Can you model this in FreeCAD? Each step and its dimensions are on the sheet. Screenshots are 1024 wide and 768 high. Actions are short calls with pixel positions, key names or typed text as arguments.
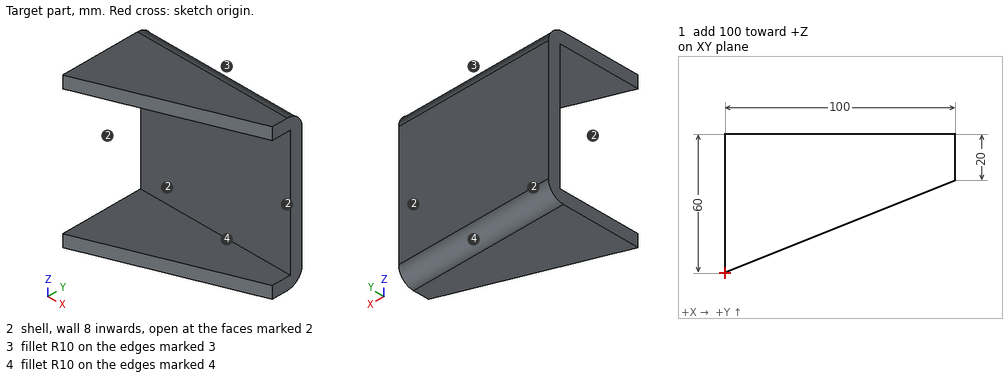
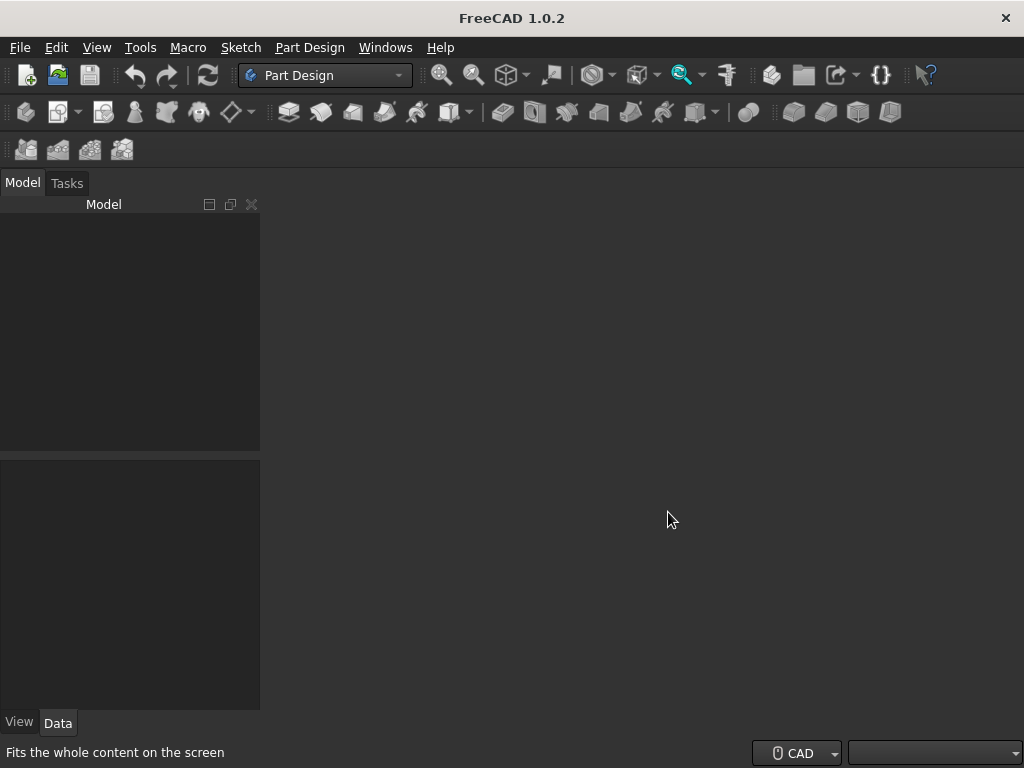
click(26, 76)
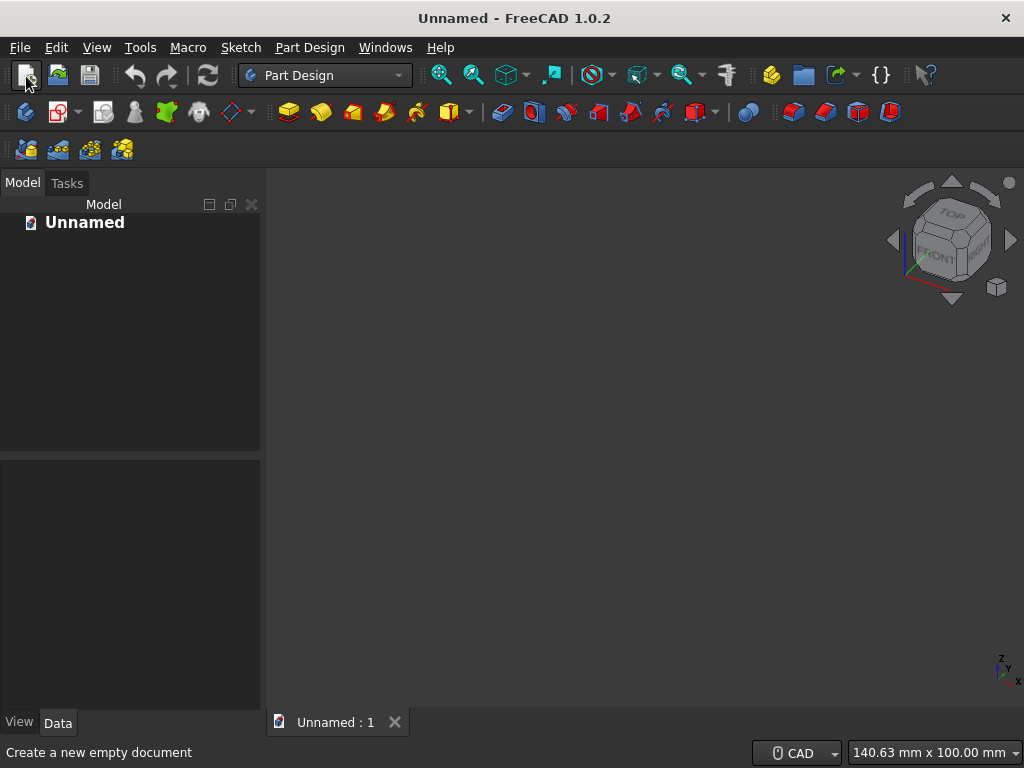
click(58, 112)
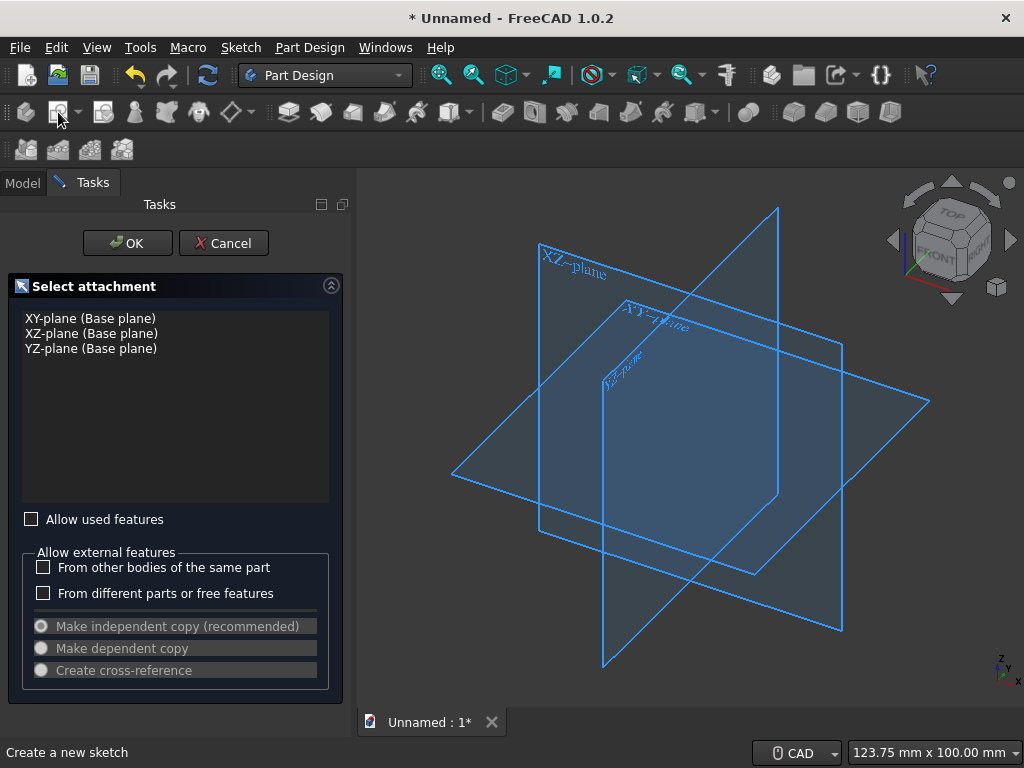
click(82, 318)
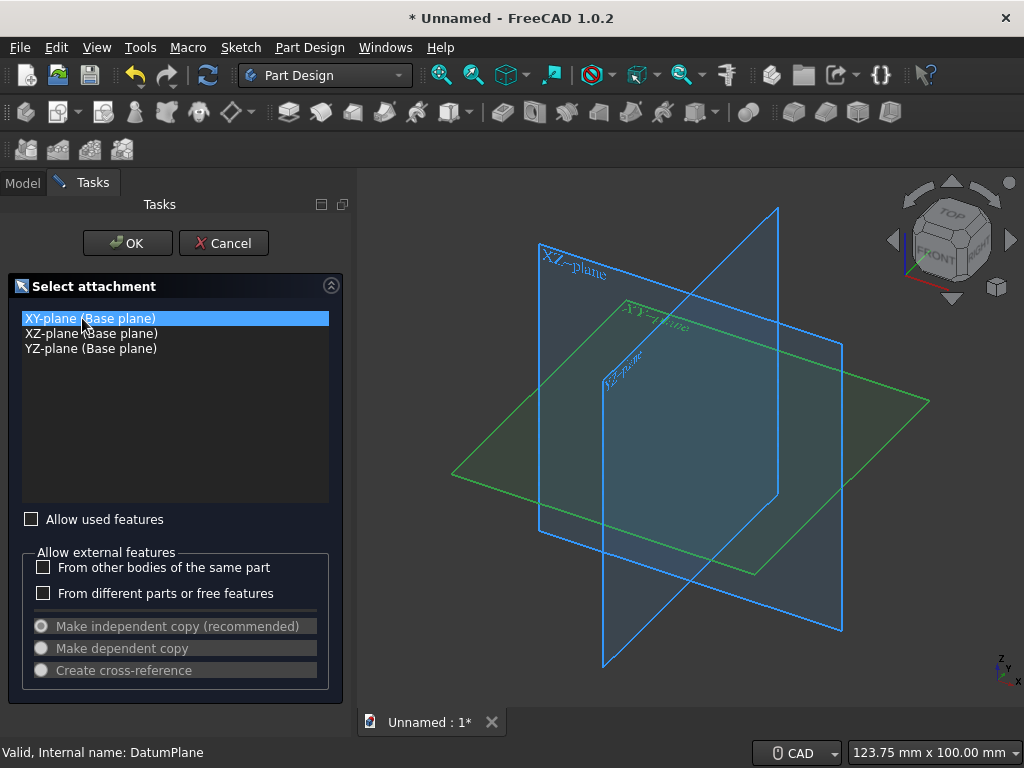
click(128, 243)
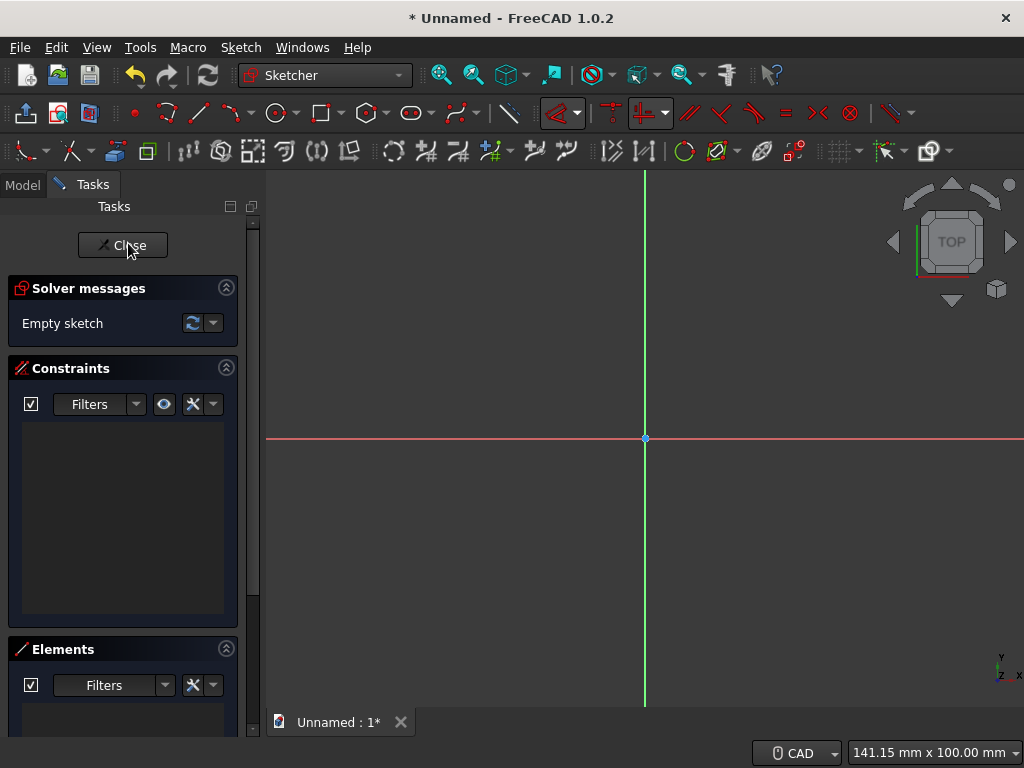
scroll(294, 634, down, 3)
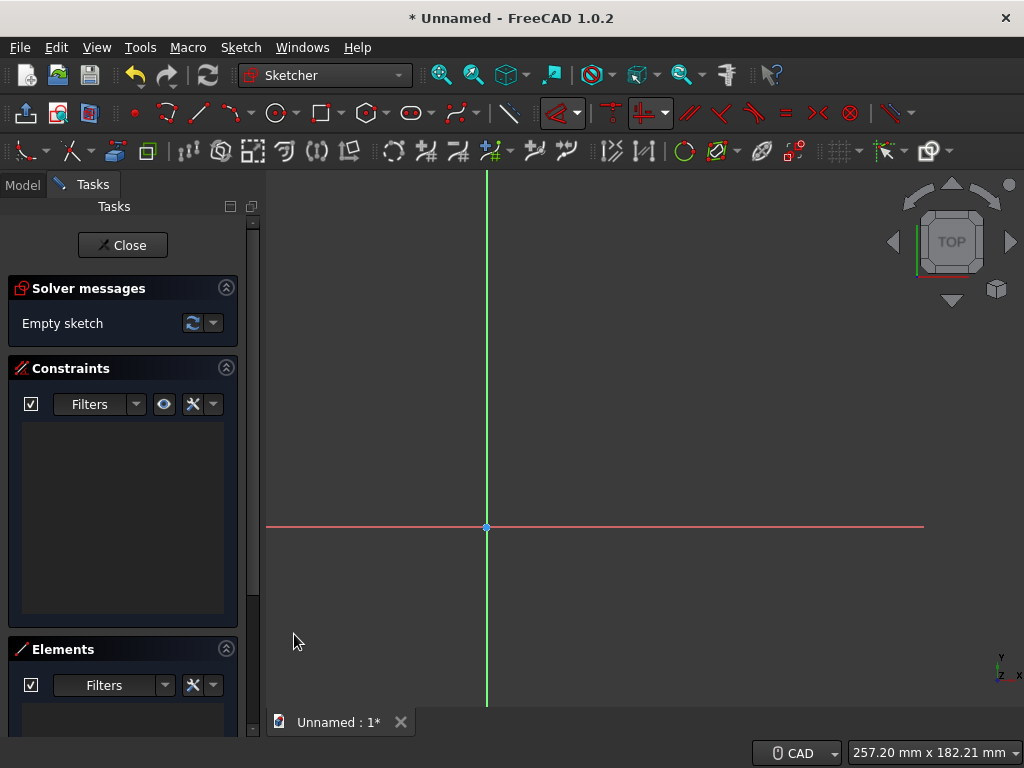
scroll(751, 439, up, 2)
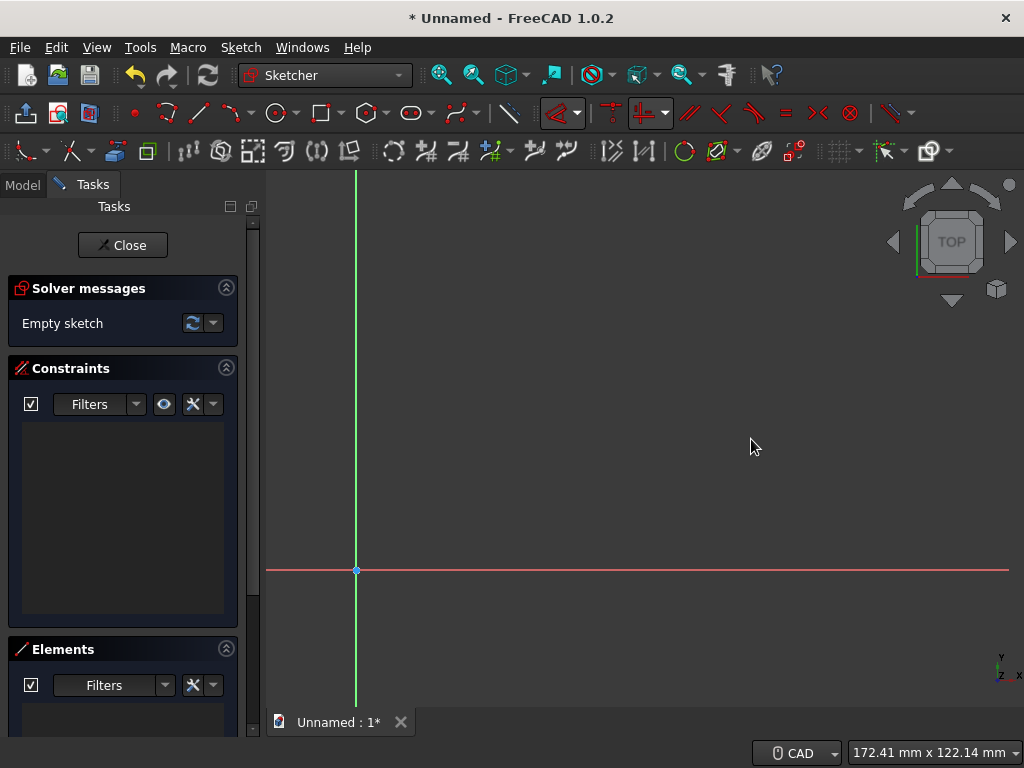
click(168, 114)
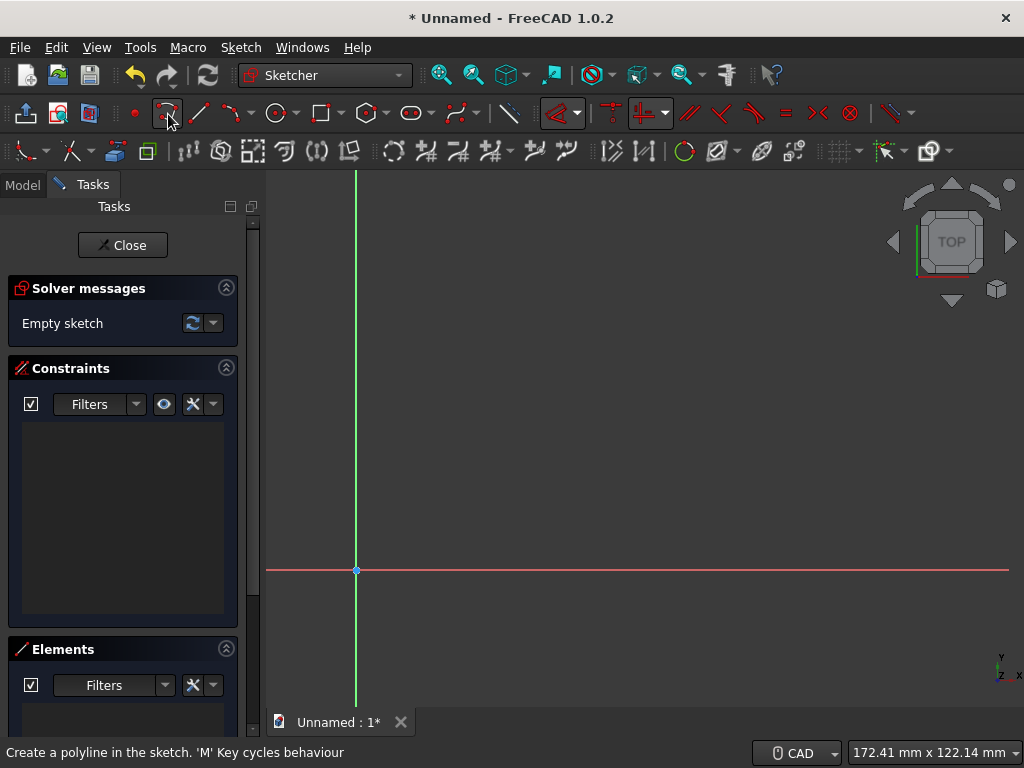
click(356, 570)
click(796, 394)
click(796, 306)
click(365, 306)
click(356, 570)
key(Escape)
key(Escape)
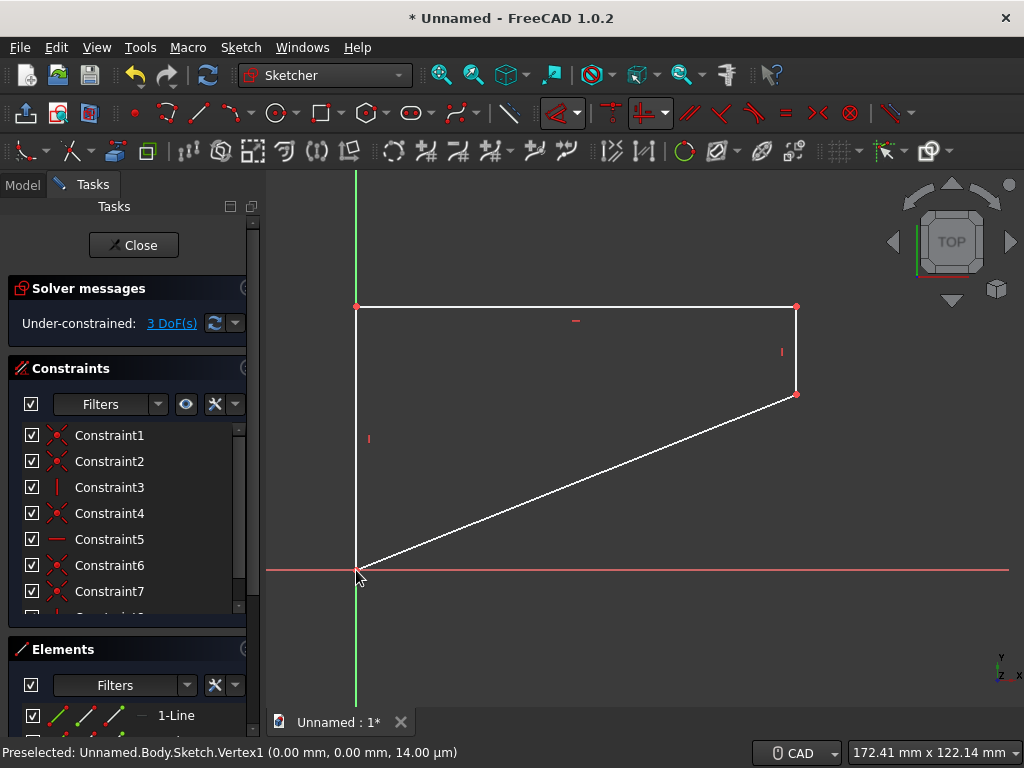
click(556, 114)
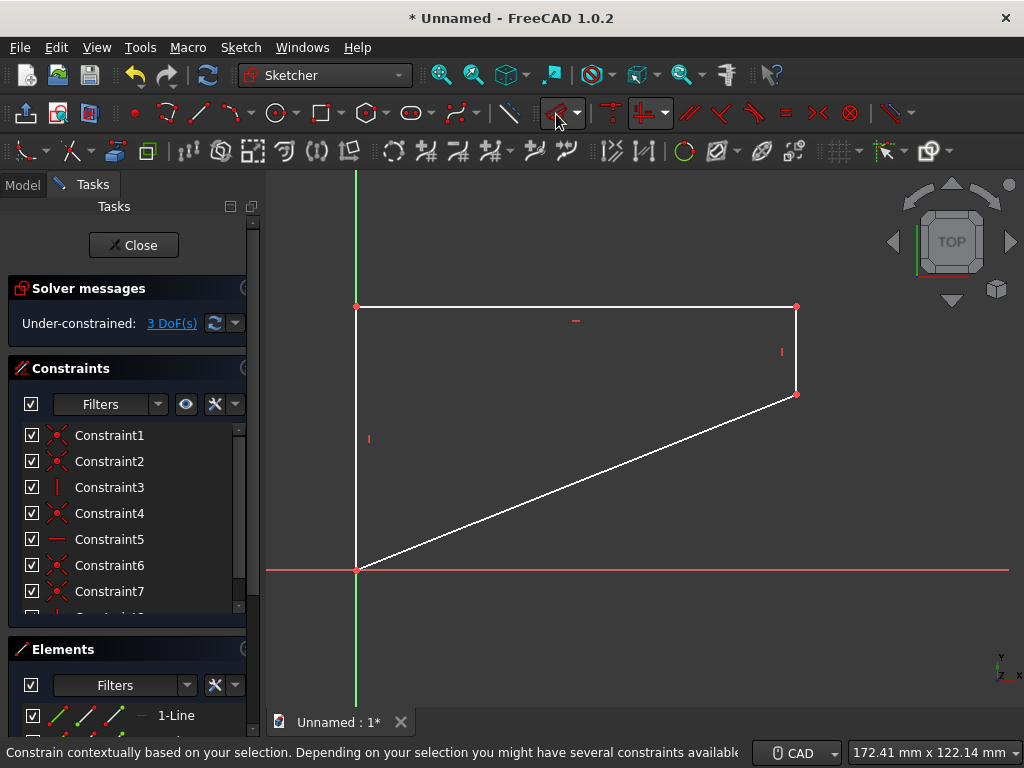
click(796, 369)
click(830, 351)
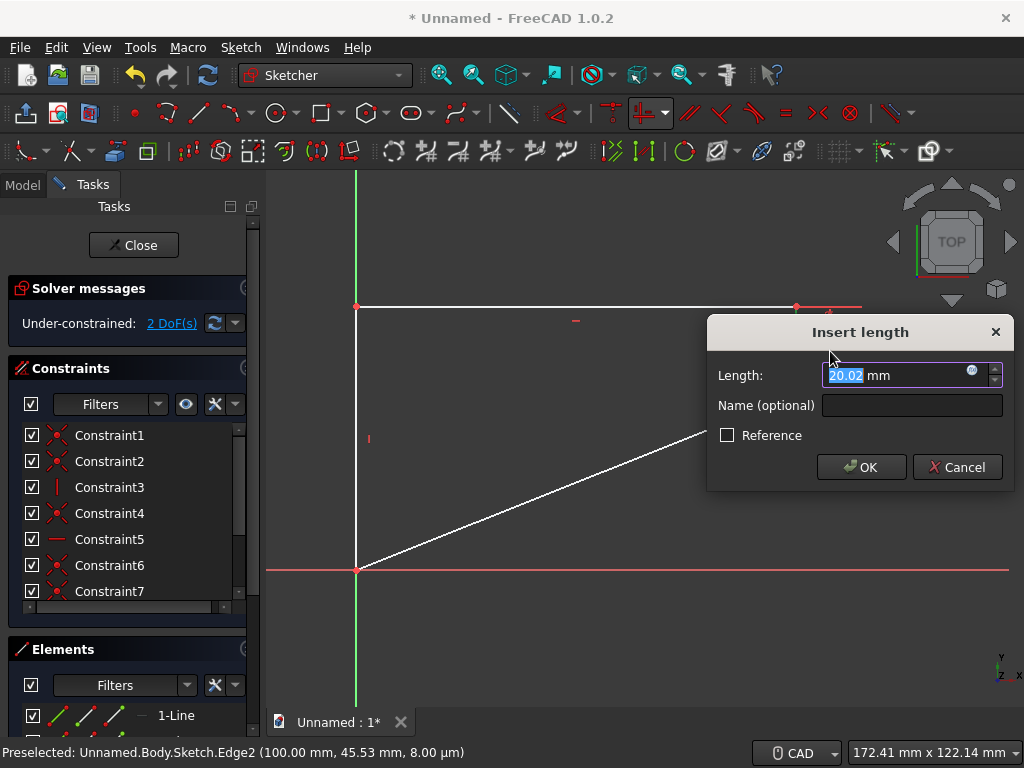
text(20)
key(Return)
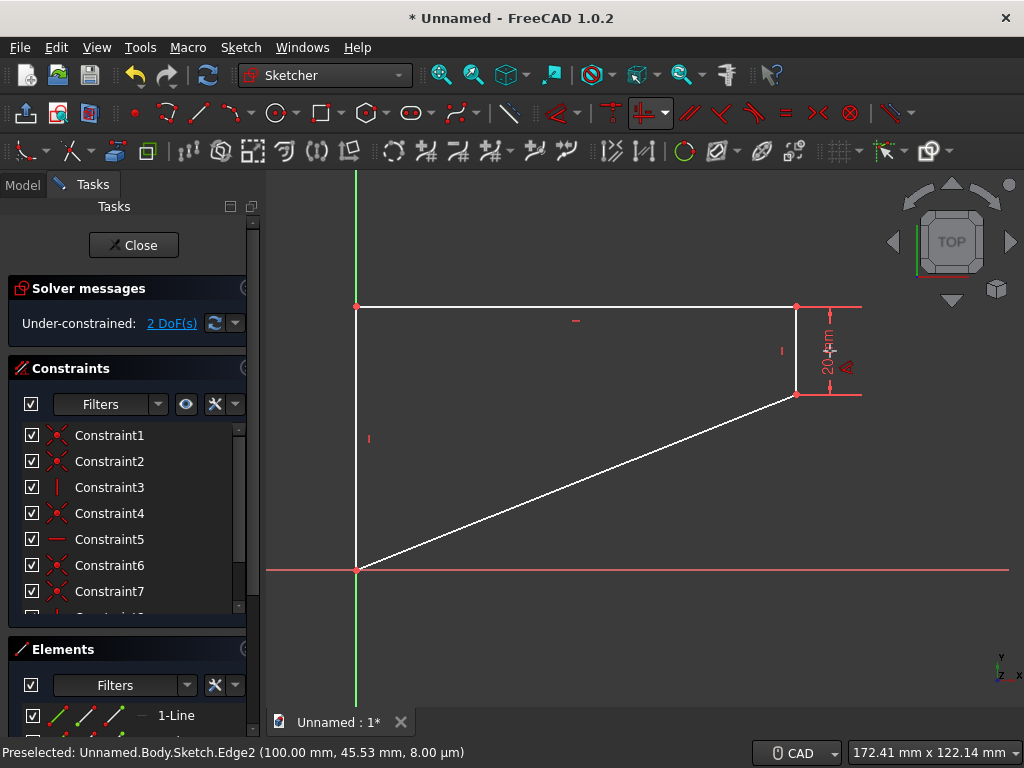
click(356, 386)
click(322, 439)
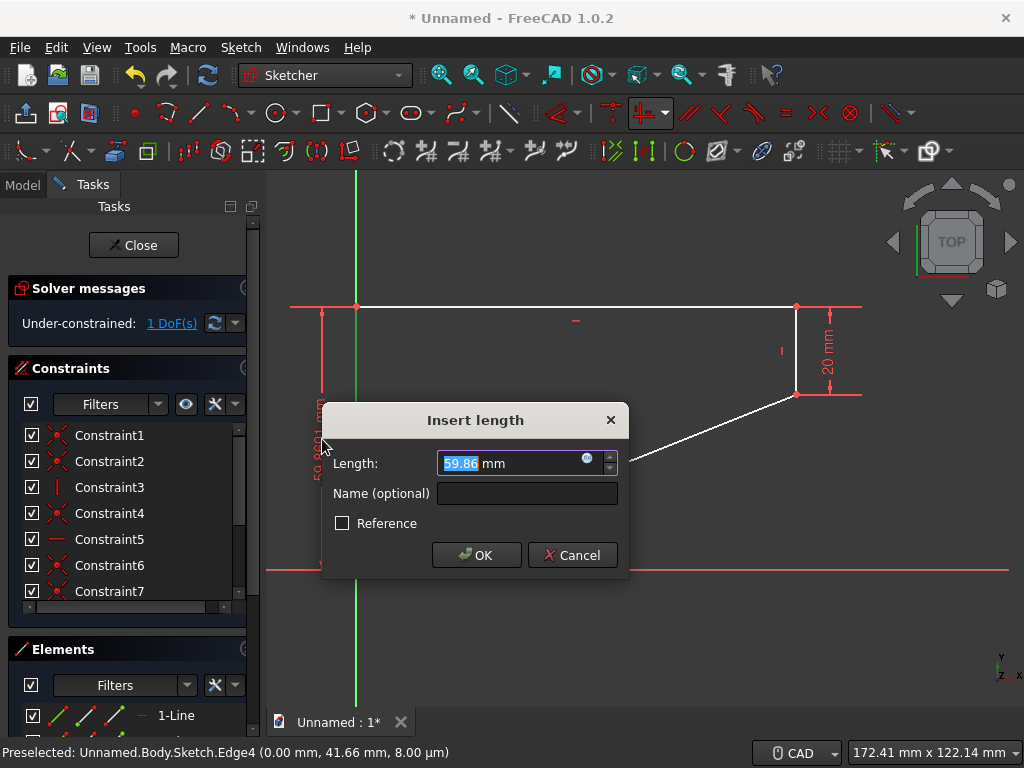
text(60)
key(Return)